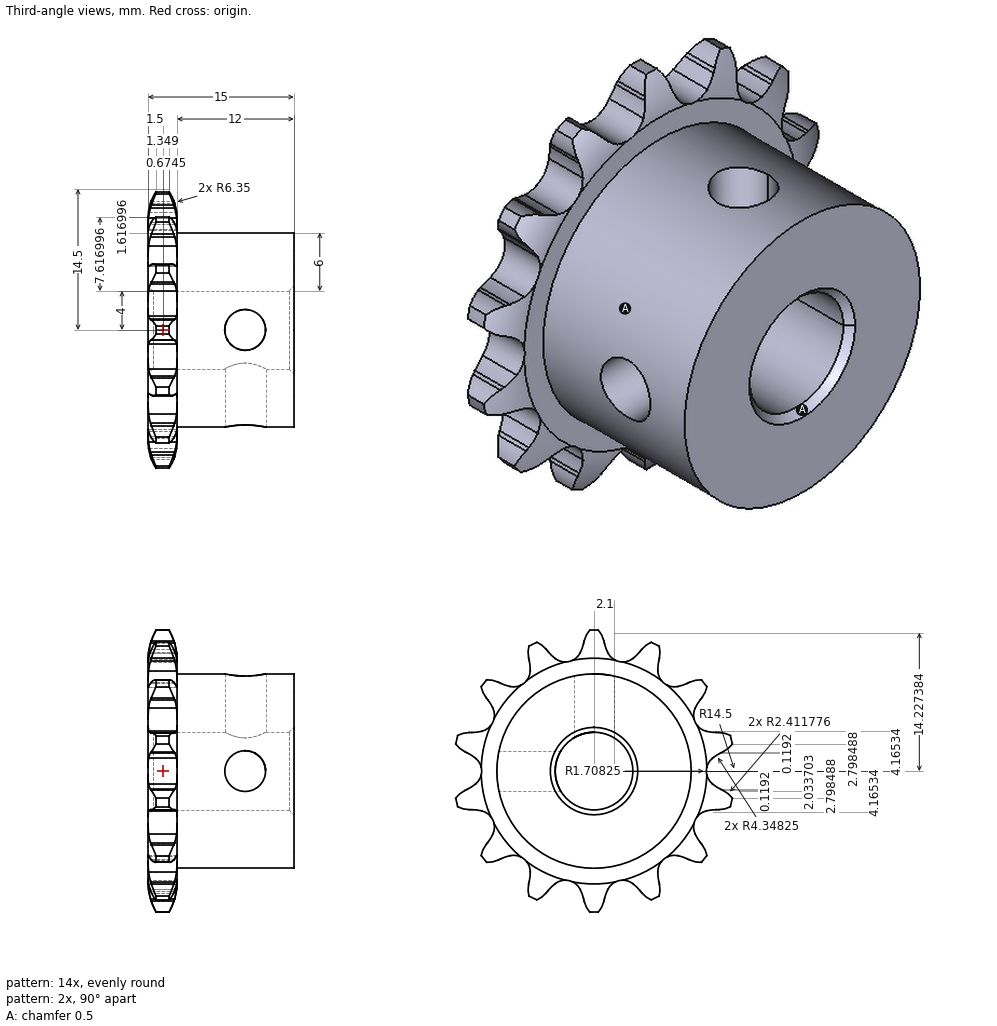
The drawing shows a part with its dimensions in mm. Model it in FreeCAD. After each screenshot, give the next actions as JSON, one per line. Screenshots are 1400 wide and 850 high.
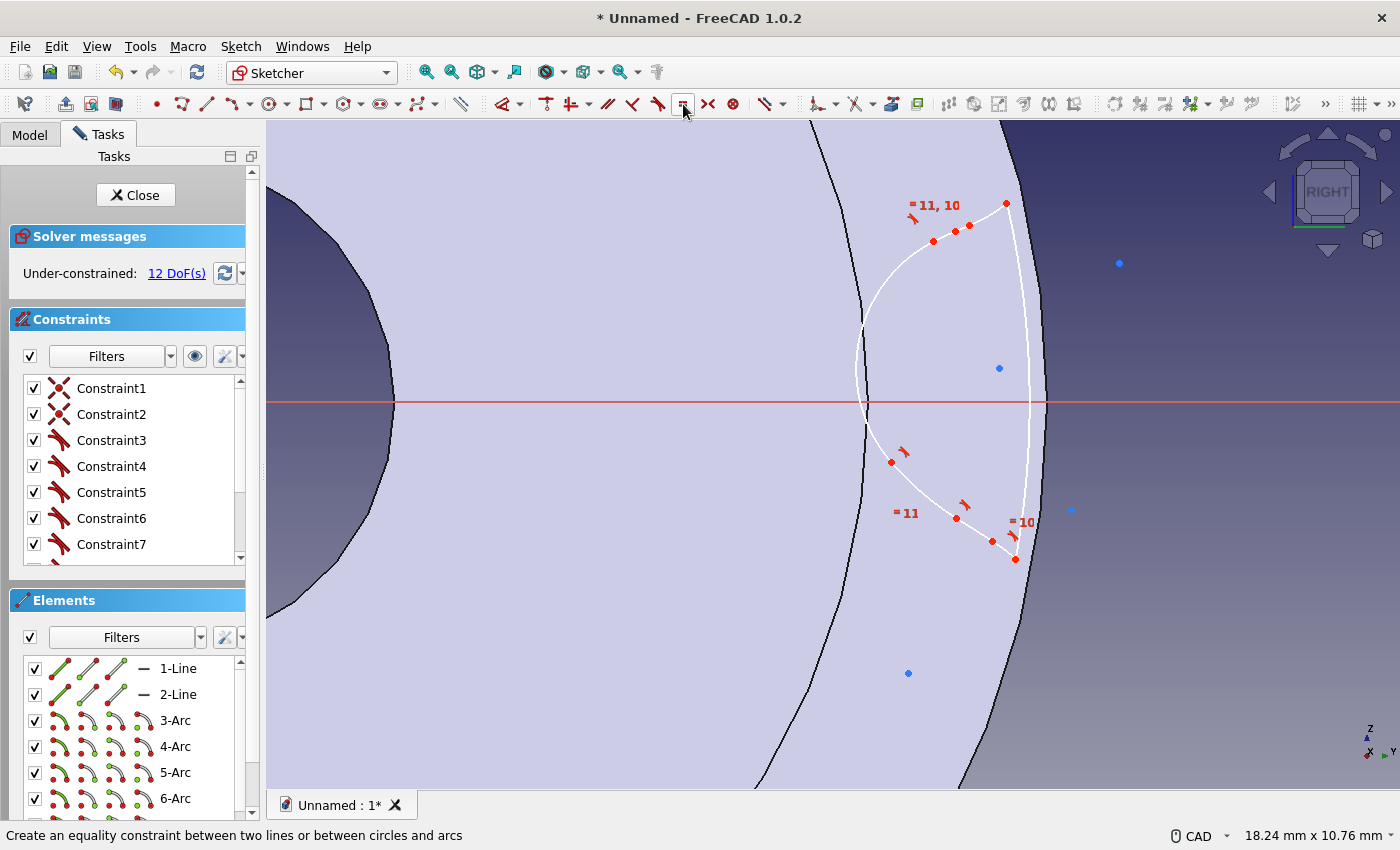
{"action": "left_click", "coordinate": [999, 369]}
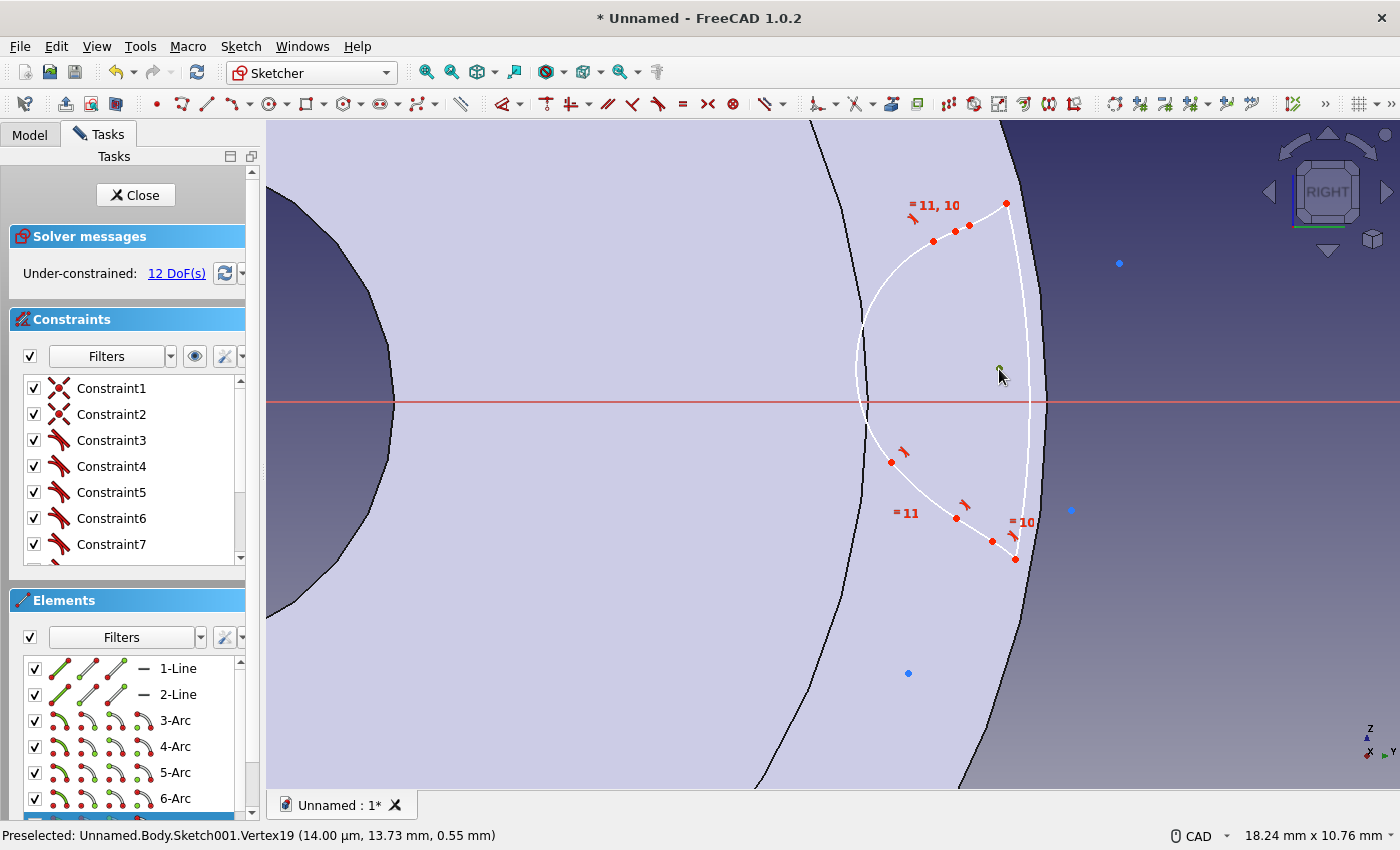
{"action": "left_click", "coordinate": [361, 402]}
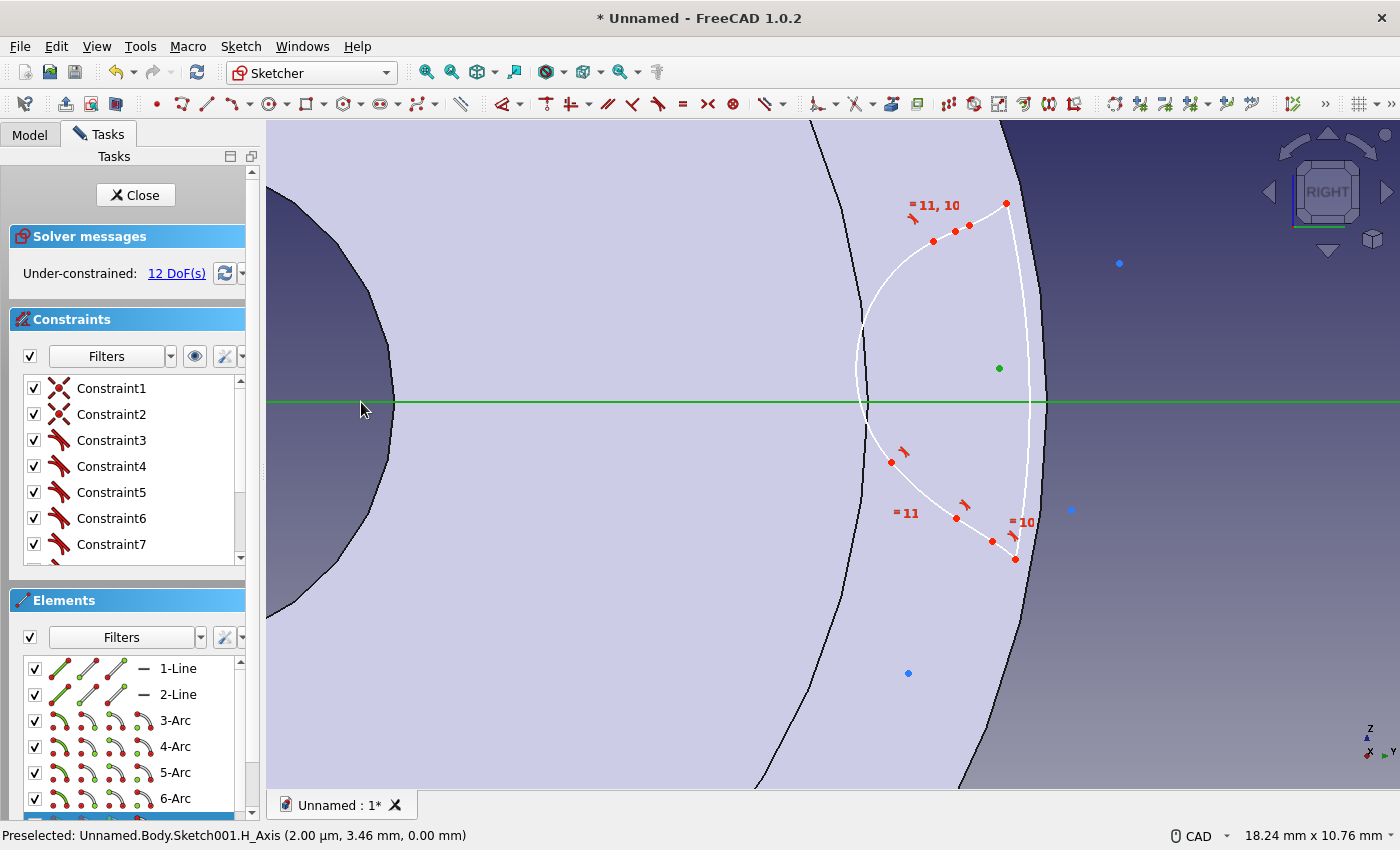
{"action": "left_click", "coordinate": [546, 104]}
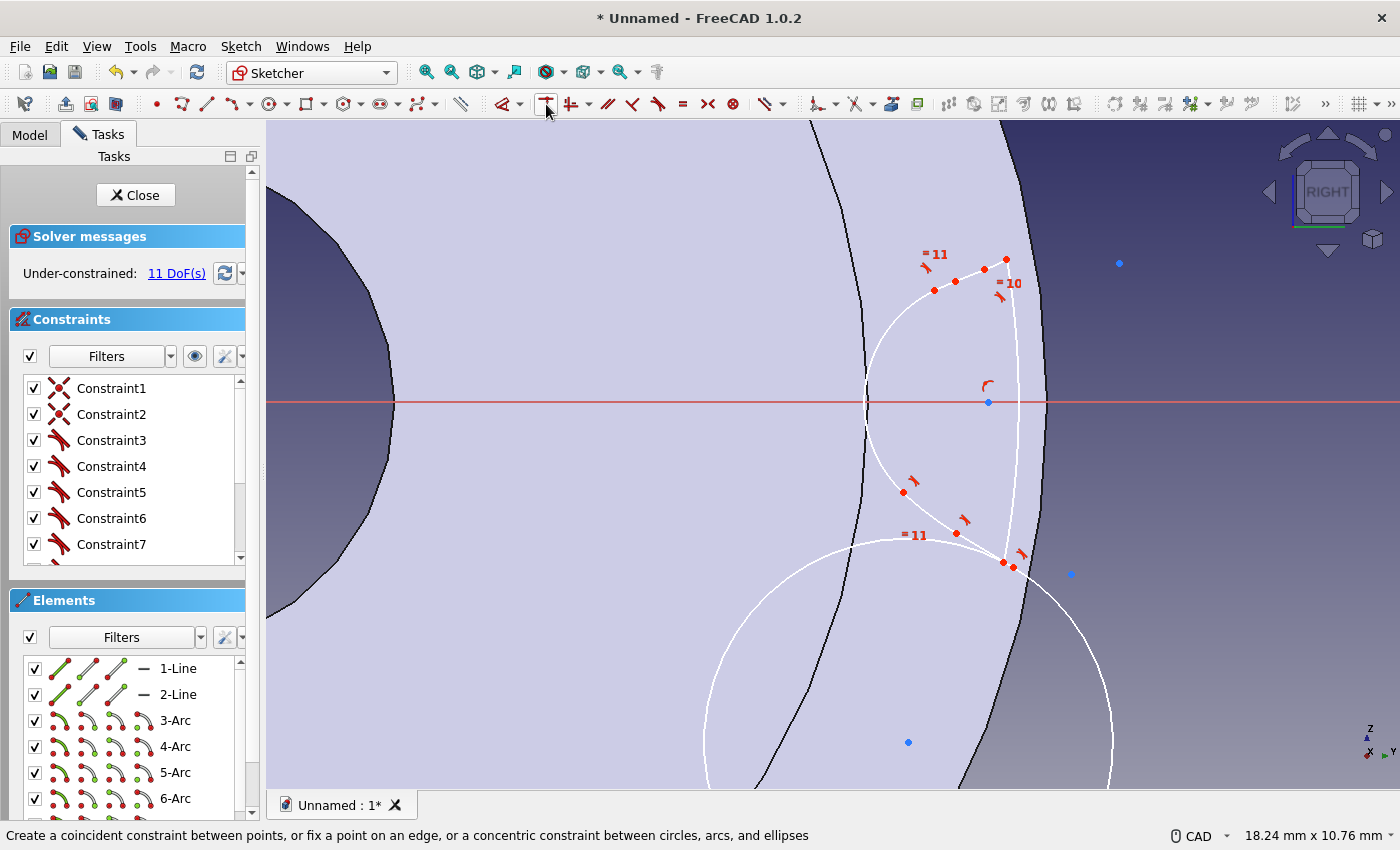
{"action": "left_click", "coordinate": [502, 104]}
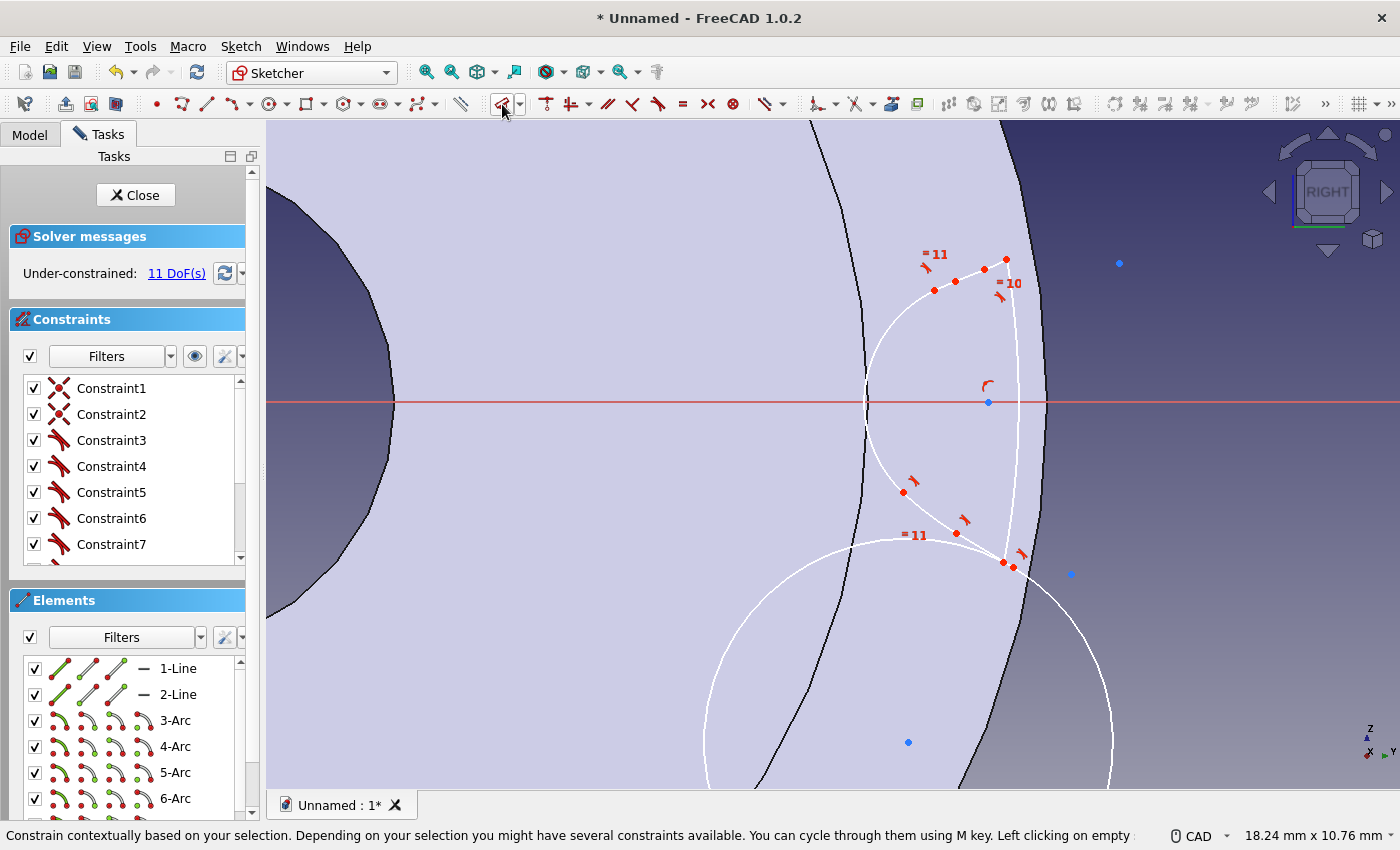
{"action": "left_click", "coordinate": [708, 705]}
{"action": "left_click", "coordinate": [677, 699]}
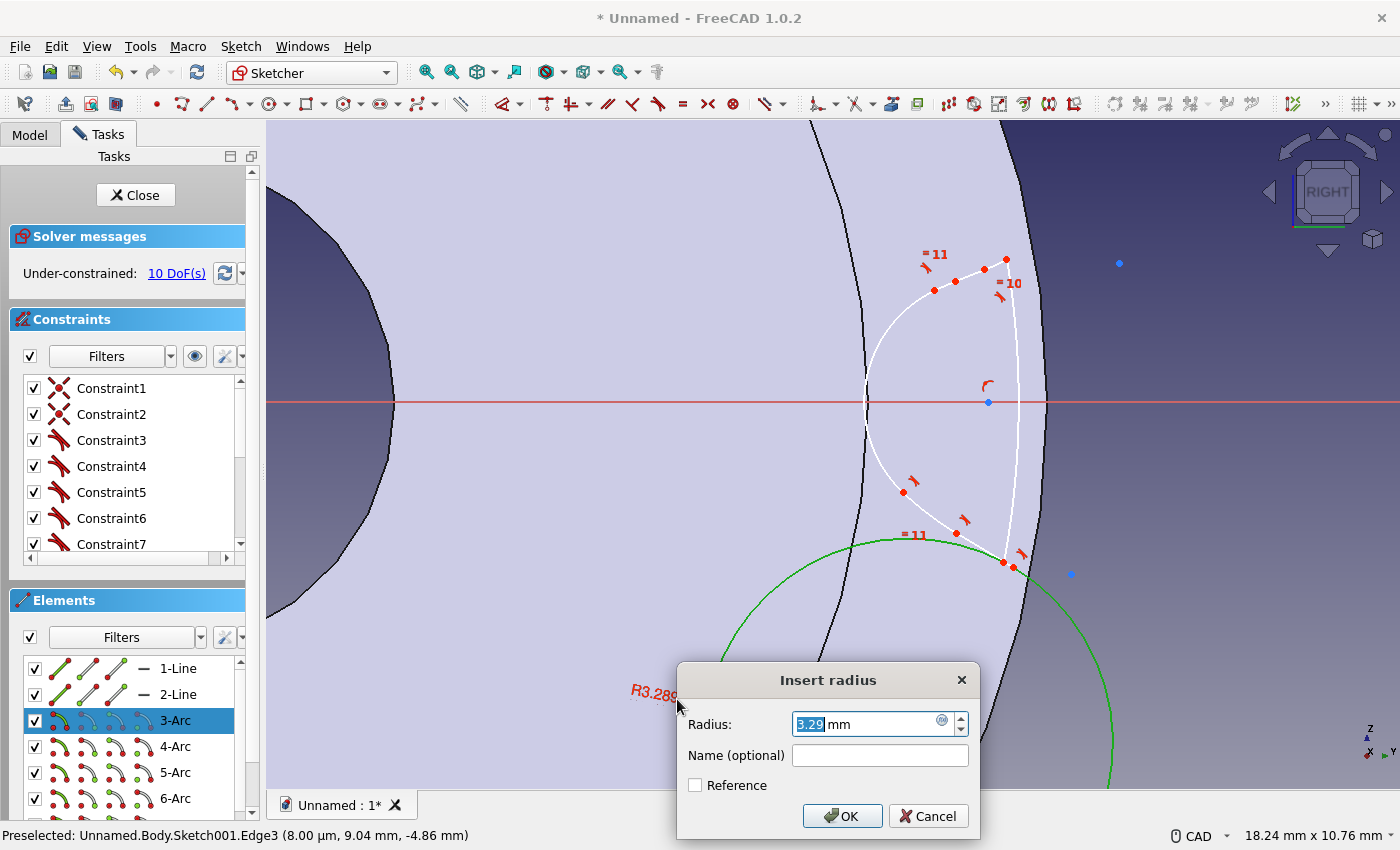
{"action": "type", "text": "2.411776"}
{"action": "key", "text": "Return"}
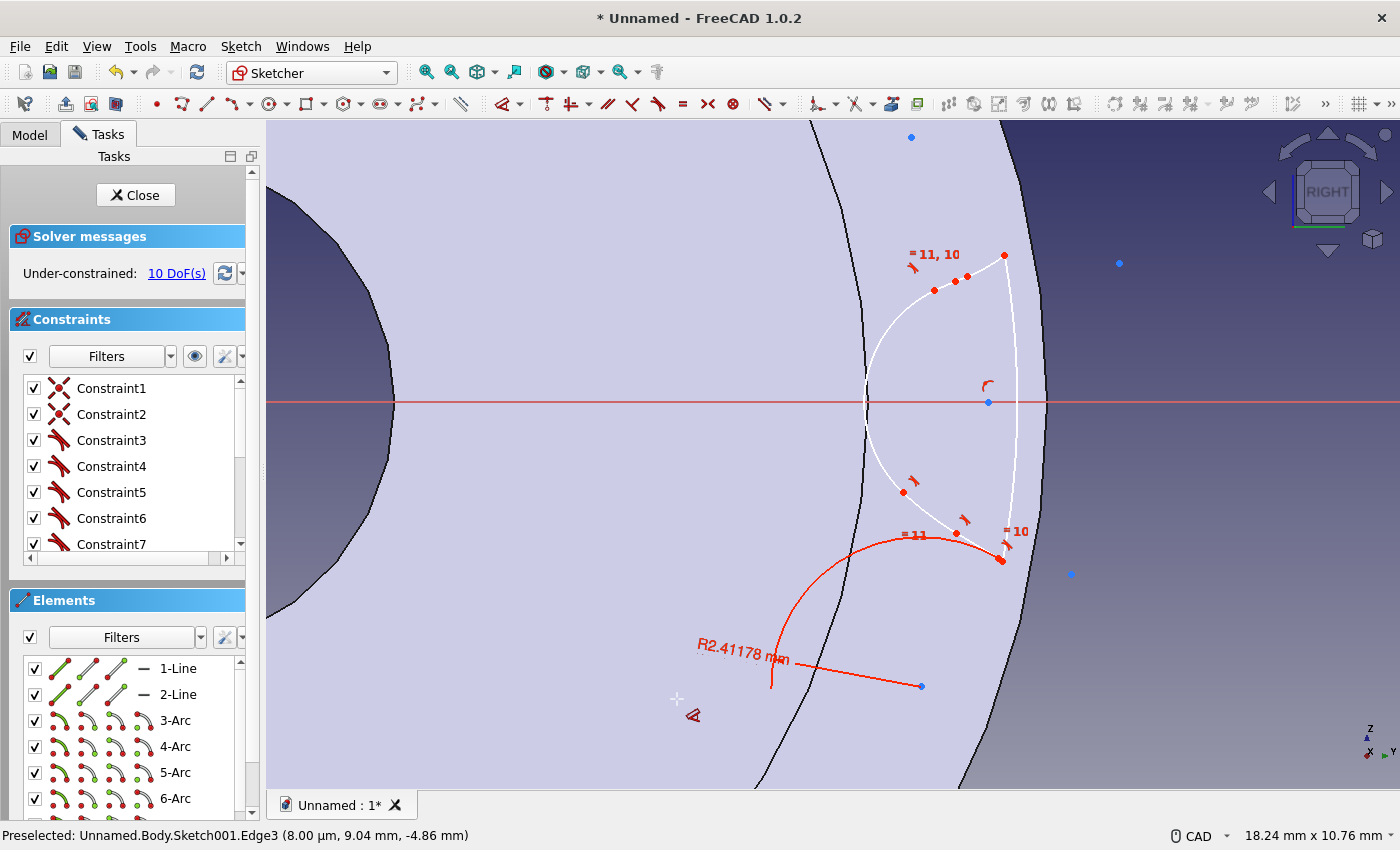
{"action": "left_click", "coordinate": [1015, 470]}
{"action": "left_click", "coordinate": [1047, 472]}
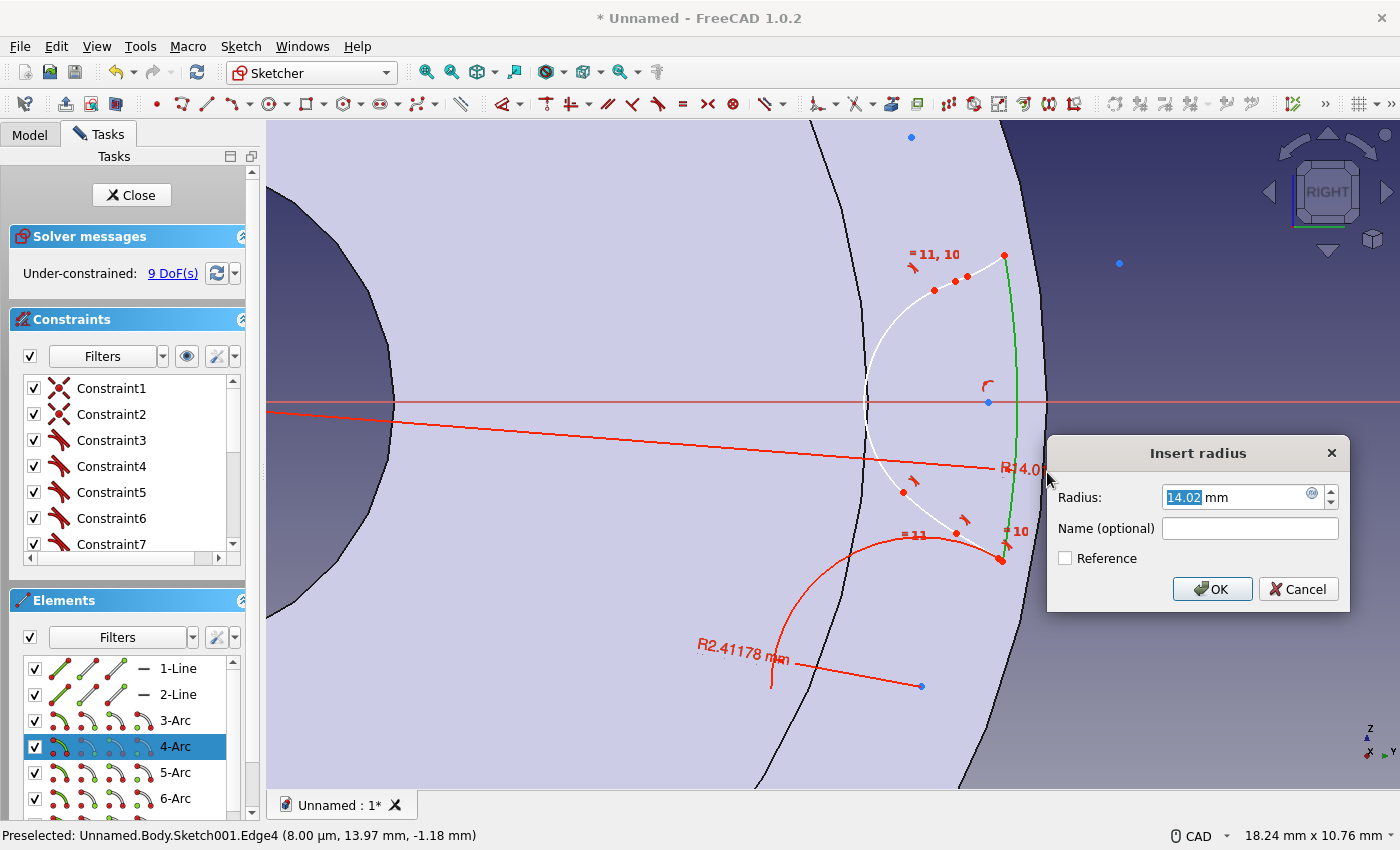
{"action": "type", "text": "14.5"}
{"action": "key", "text": "Return"}